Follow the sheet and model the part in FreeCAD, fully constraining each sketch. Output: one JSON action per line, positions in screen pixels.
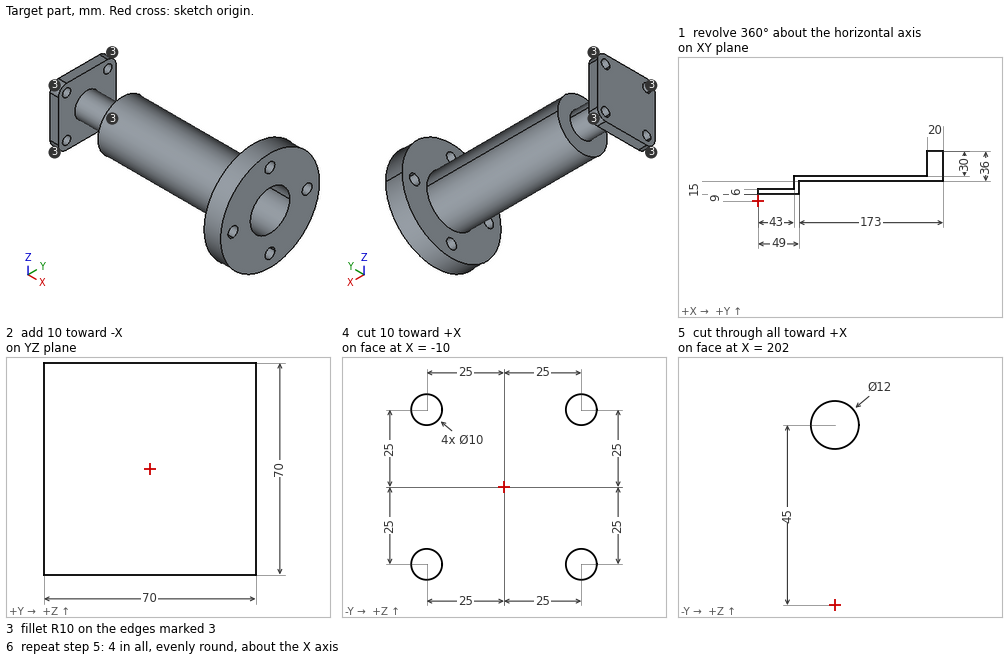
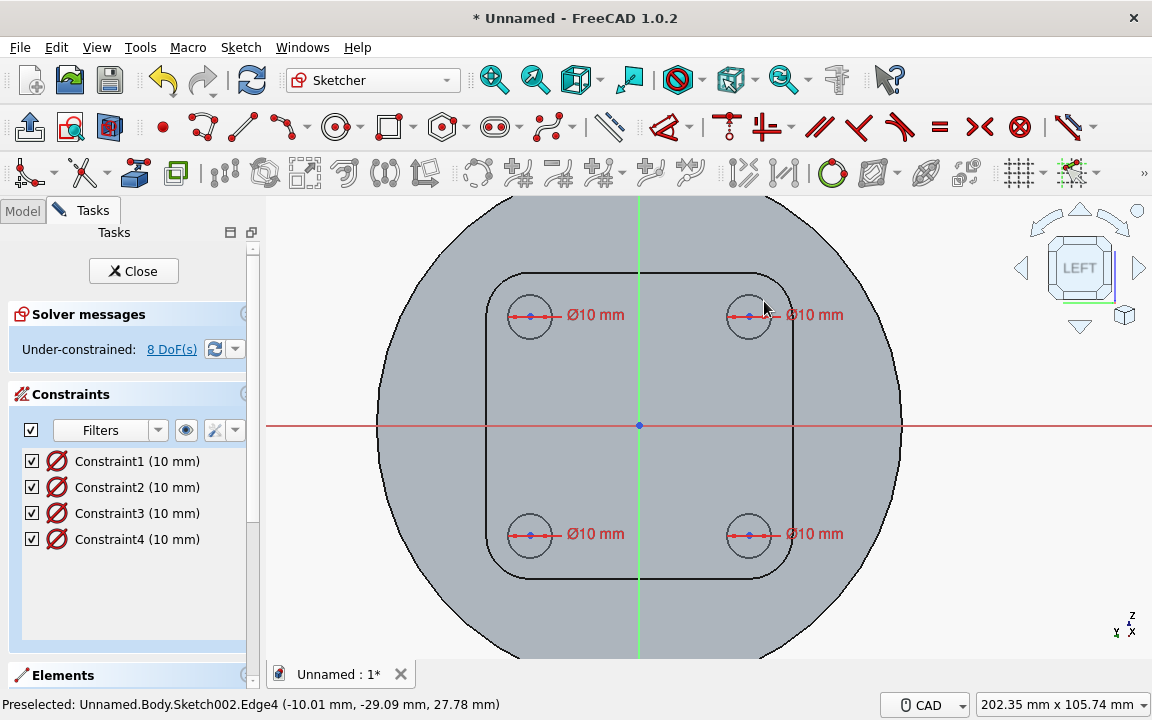
{"action": "key", "text": "d"}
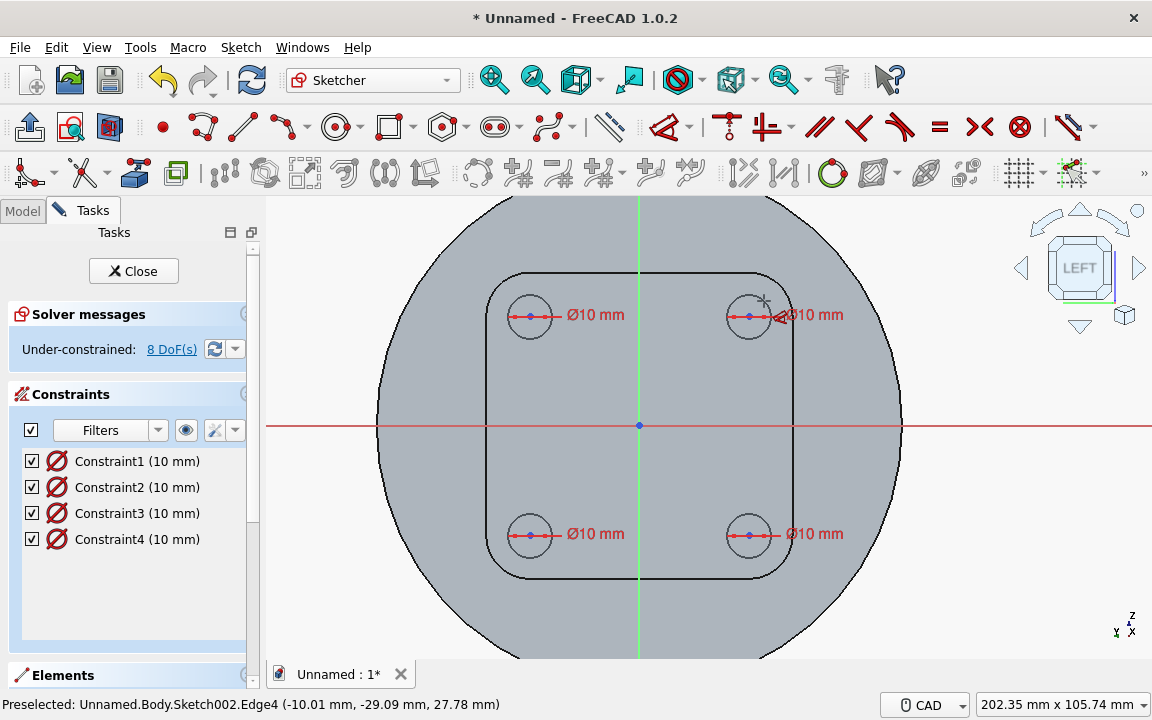
{"action": "left_click", "coordinate": [530, 317]}
{"action": "left_click", "coordinate": [585, 283]}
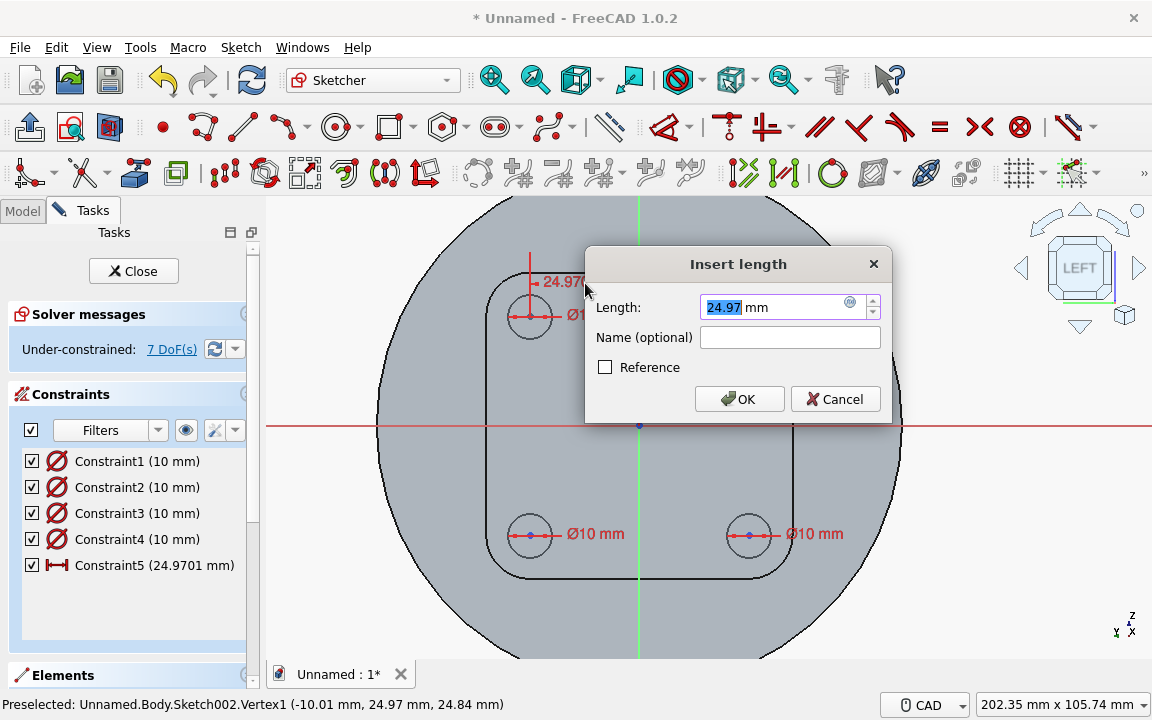
{"action": "type", "text": "25"}
{"action": "key", "text": "Return"}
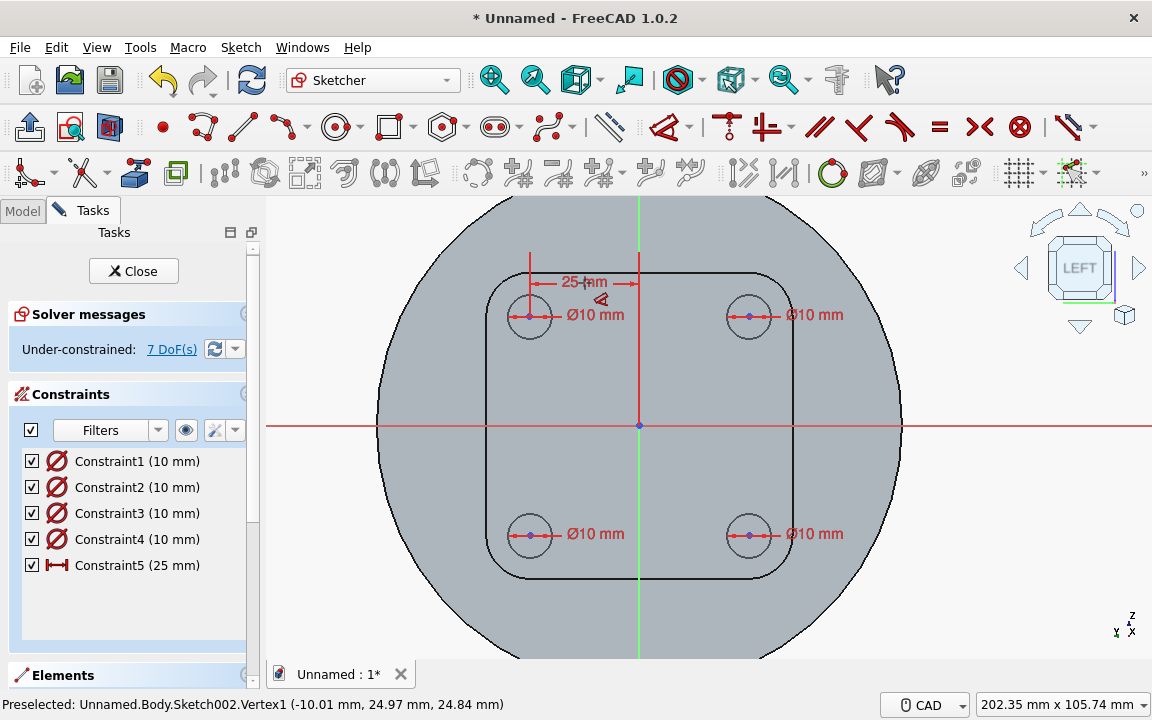
{"action": "left_click", "coordinate": [530, 317]}
{"action": "left_click", "coordinate": [496, 371]}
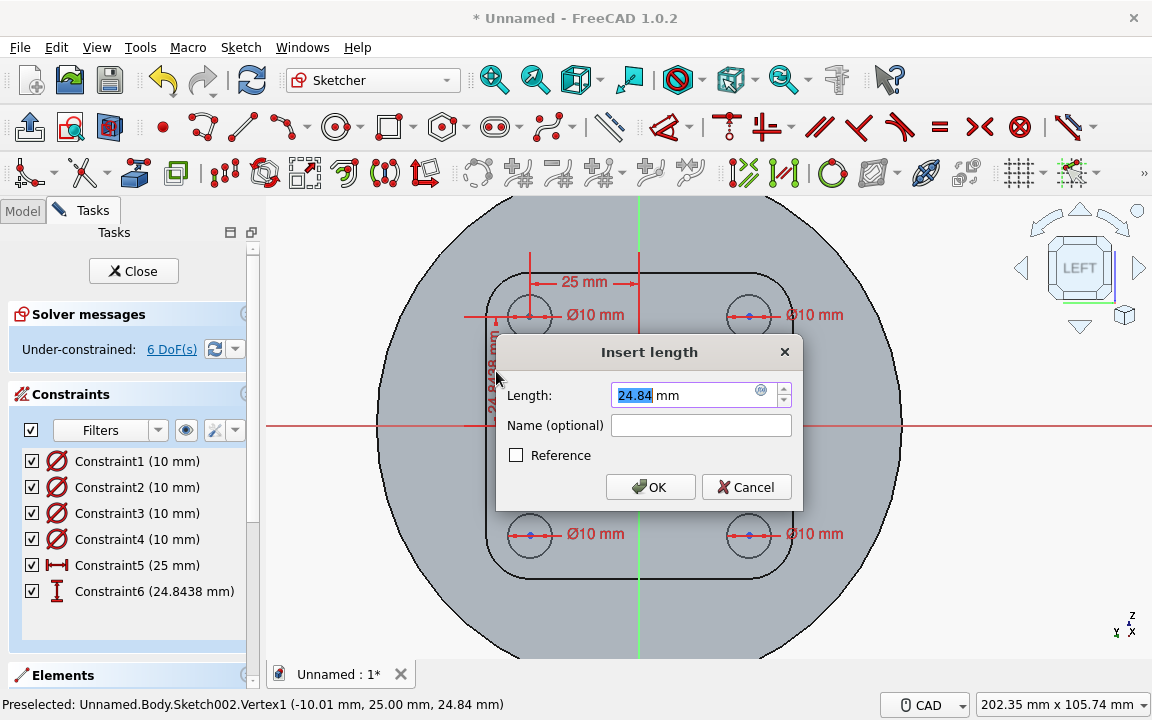
{"action": "type", "text": "25"}
{"action": "key", "text": "Return"}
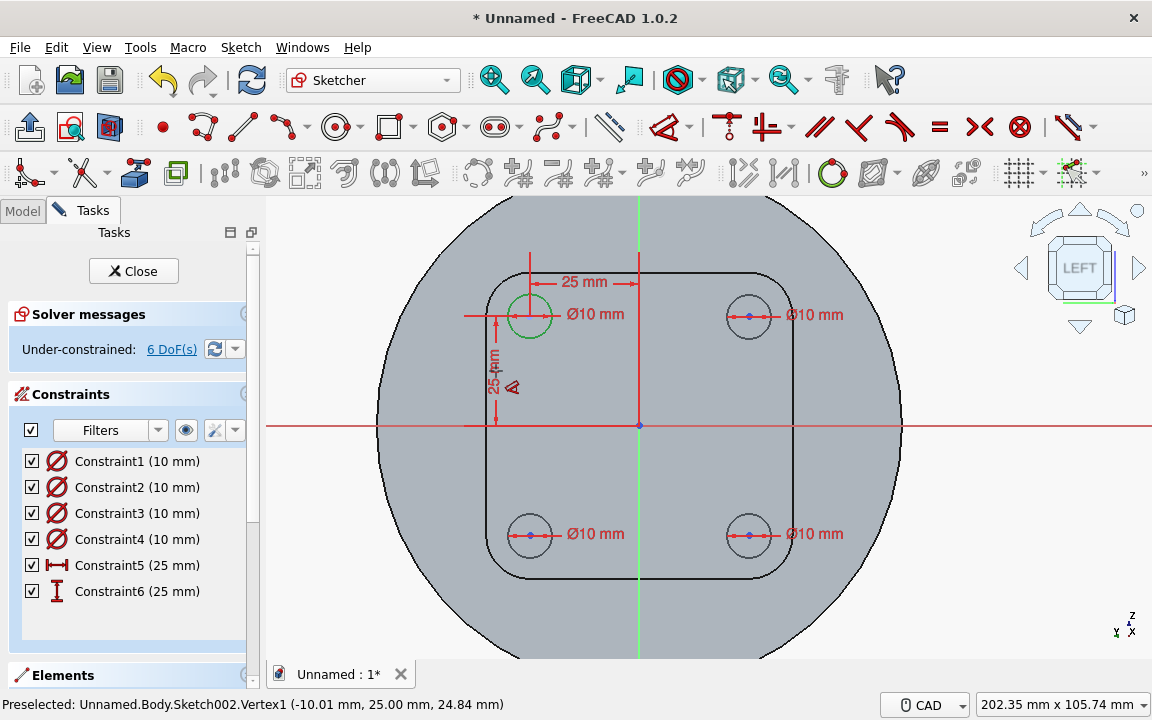
{"action": "left_click", "coordinate": [530, 536]}
{"action": "left_click", "coordinate": [585, 570]}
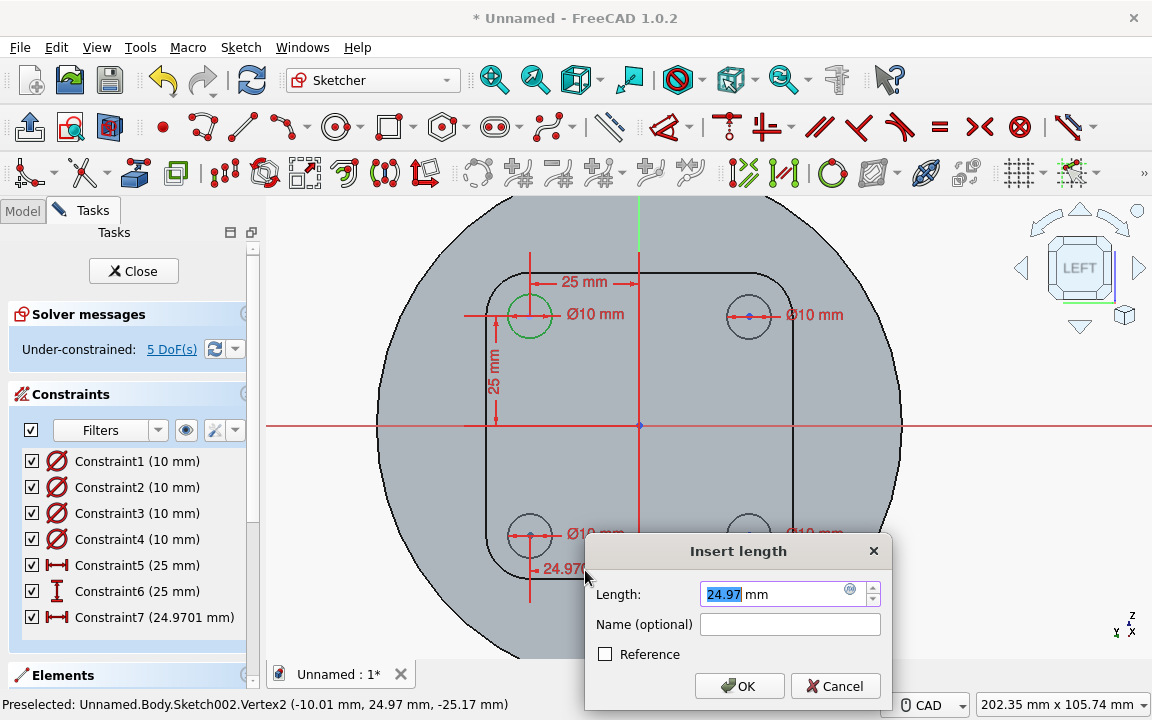
{"action": "type", "text": "25"}
{"action": "key", "text": "Return"}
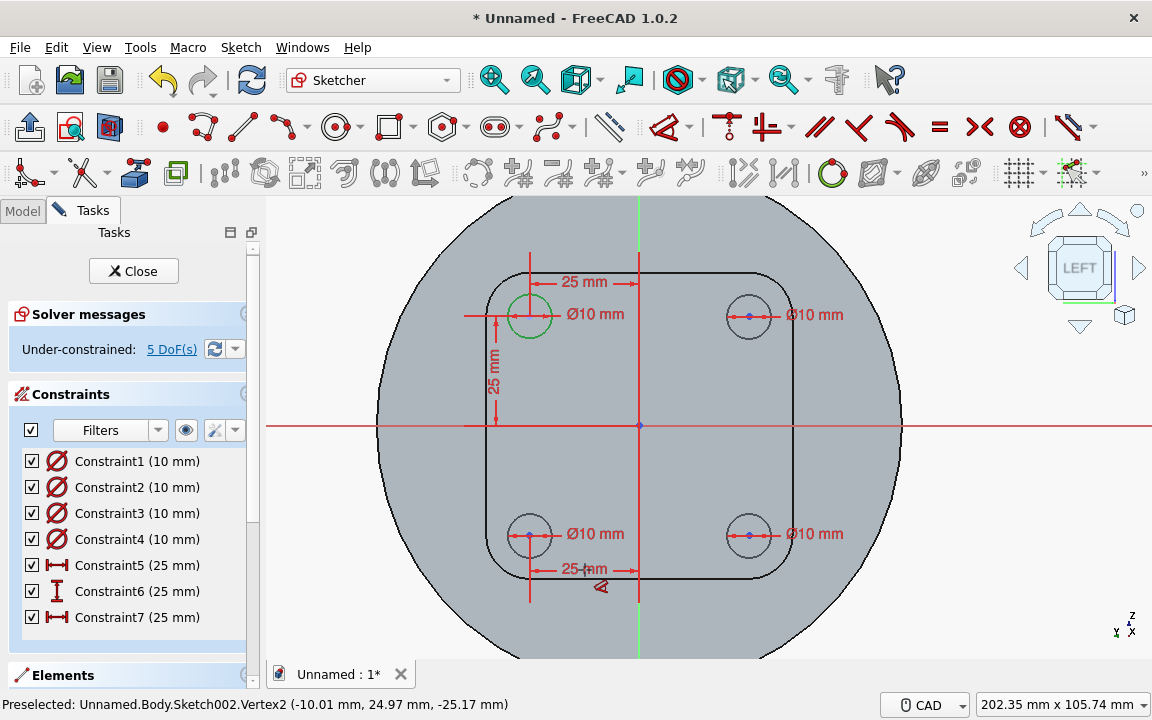
{"action": "left_click", "coordinate": [530, 536]}
{"action": "left_click", "coordinate": [496, 481]}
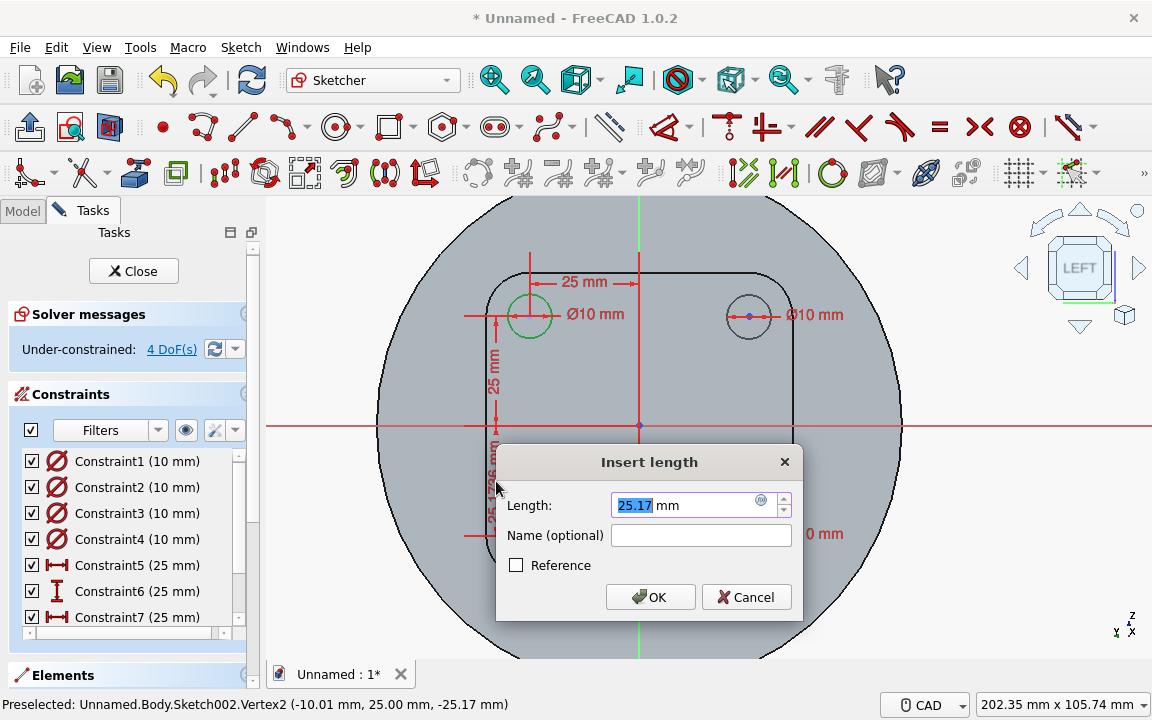
{"action": "type", "text": "25"}
{"action": "key", "text": "Return"}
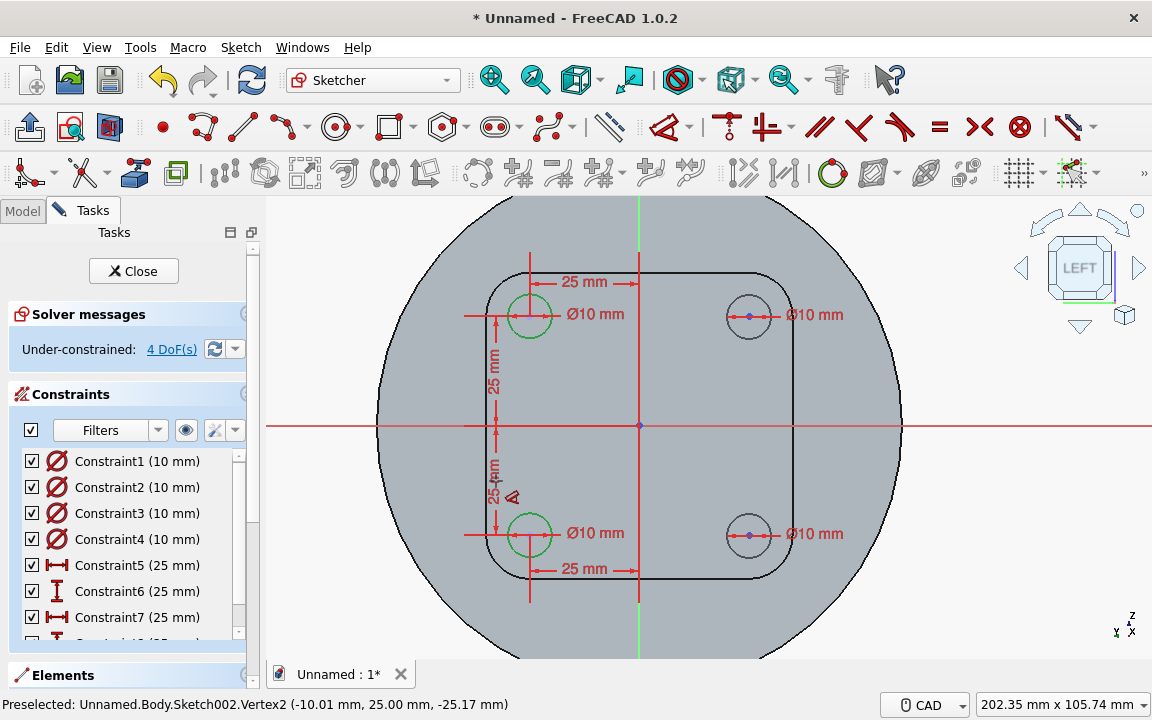
{"action": "left_click", "coordinate": [749, 536]}
{"action": "left_click", "coordinate": [694, 570]}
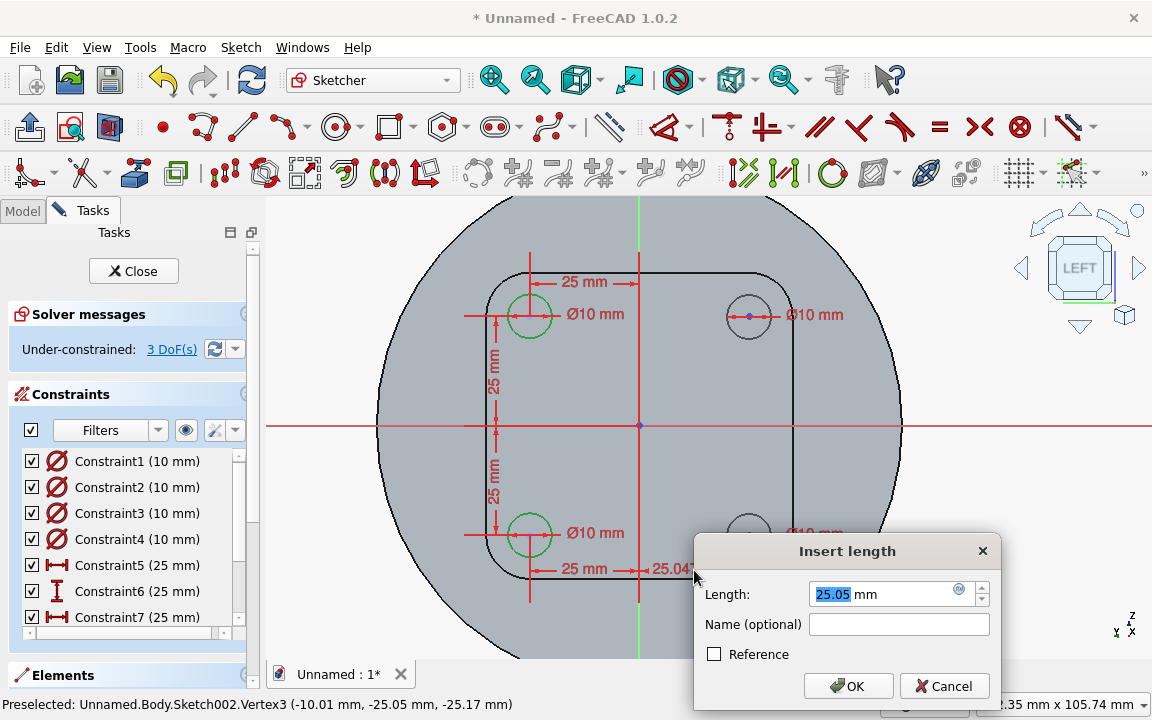
{"action": "type", "text": "25"}
{"action": "key", "text": "Return"}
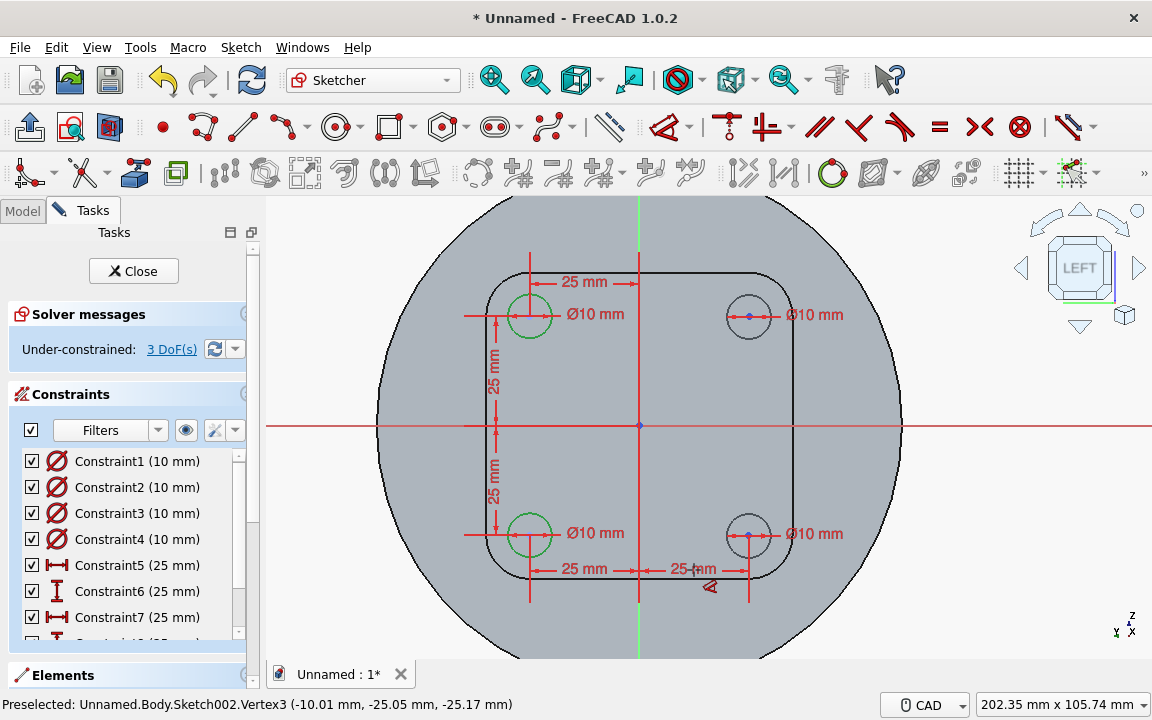
{"action": "left_click", "coordinate": [749, 536]}
{"action": "left_click", "coordinate": [783, 481]}